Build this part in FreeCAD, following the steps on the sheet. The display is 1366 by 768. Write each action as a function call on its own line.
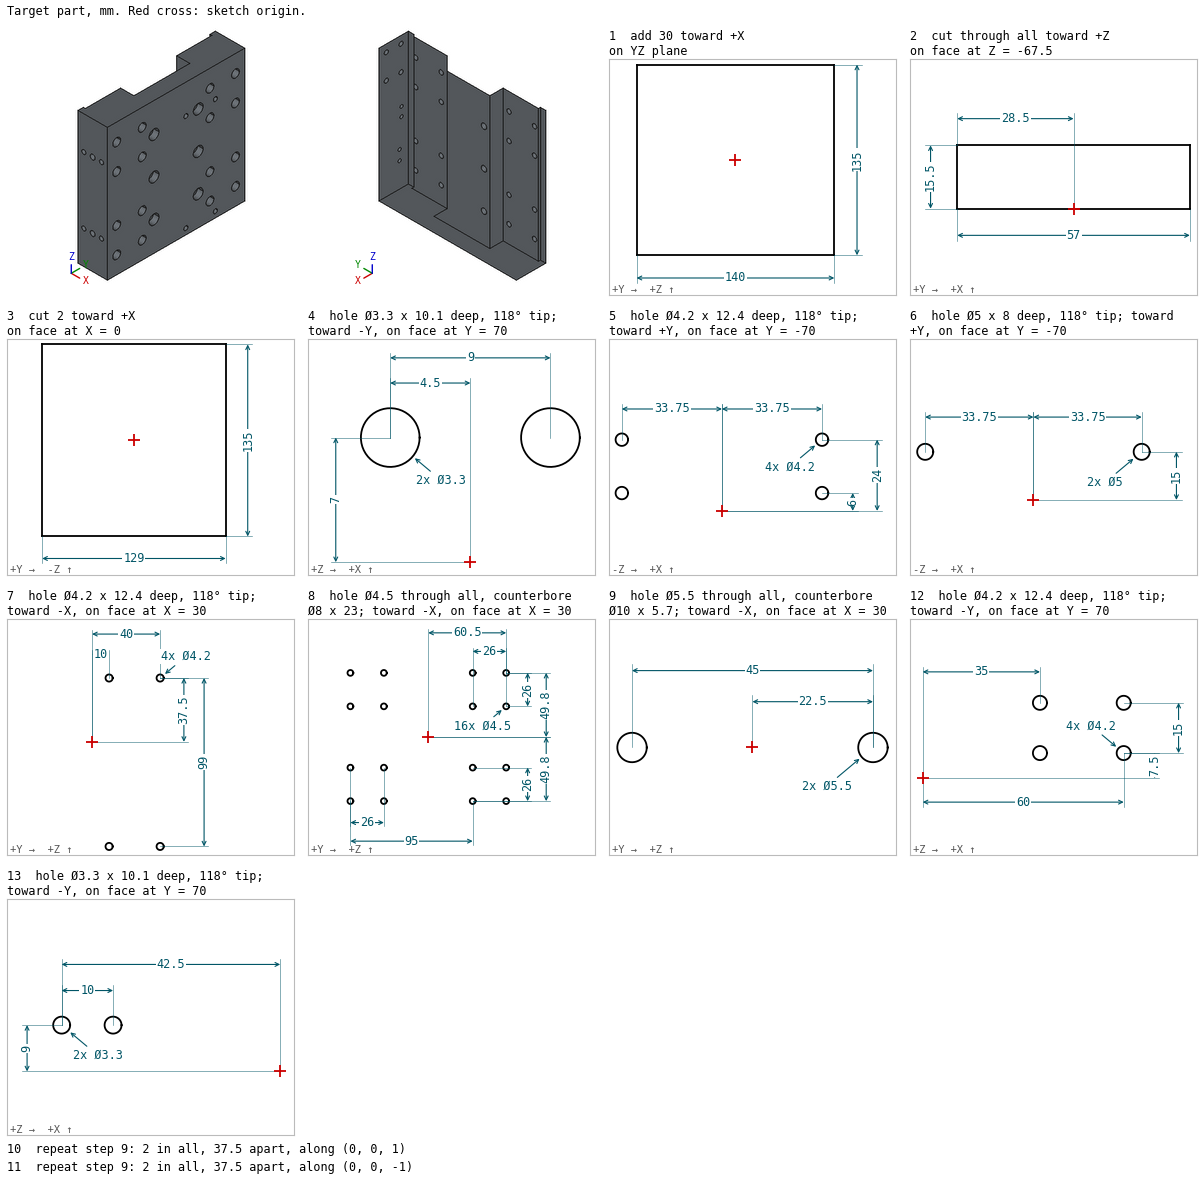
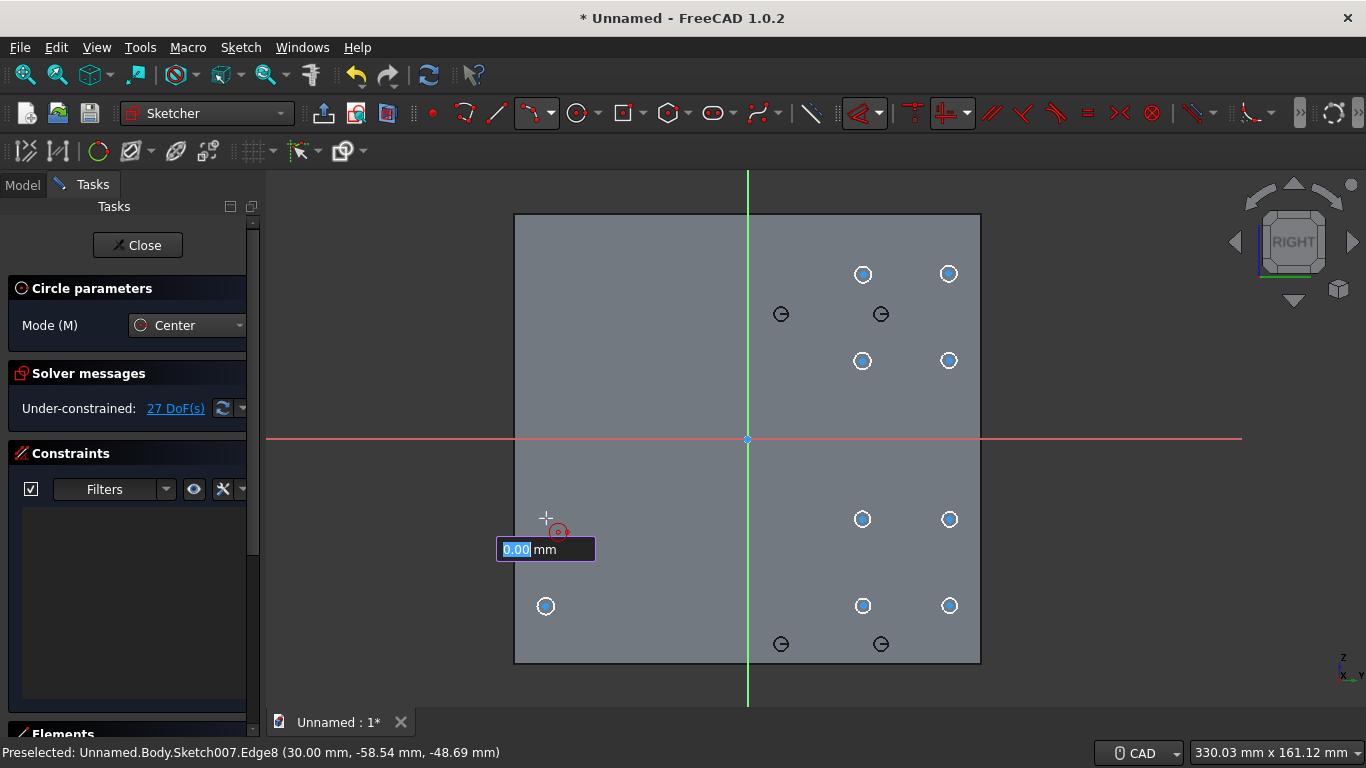
scroll(551, 513, up, 4)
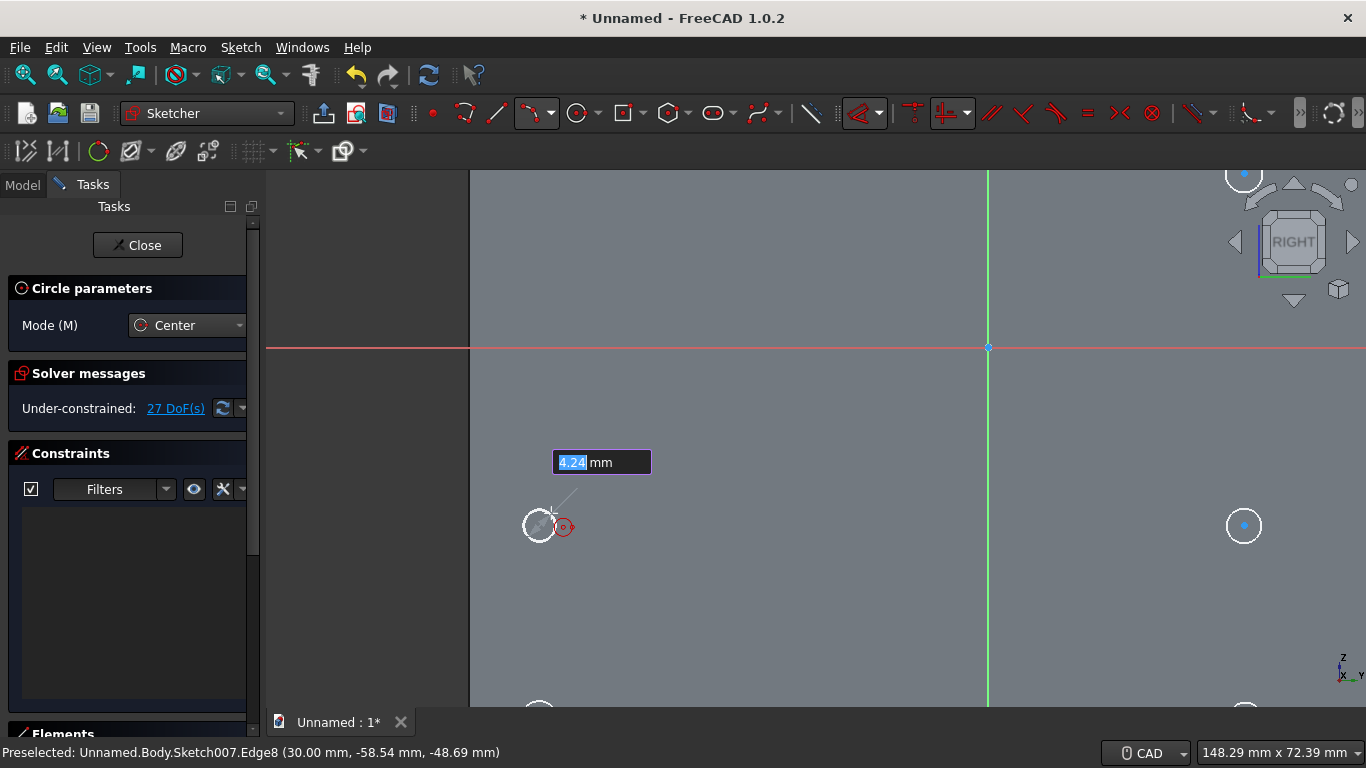
click(551, 512)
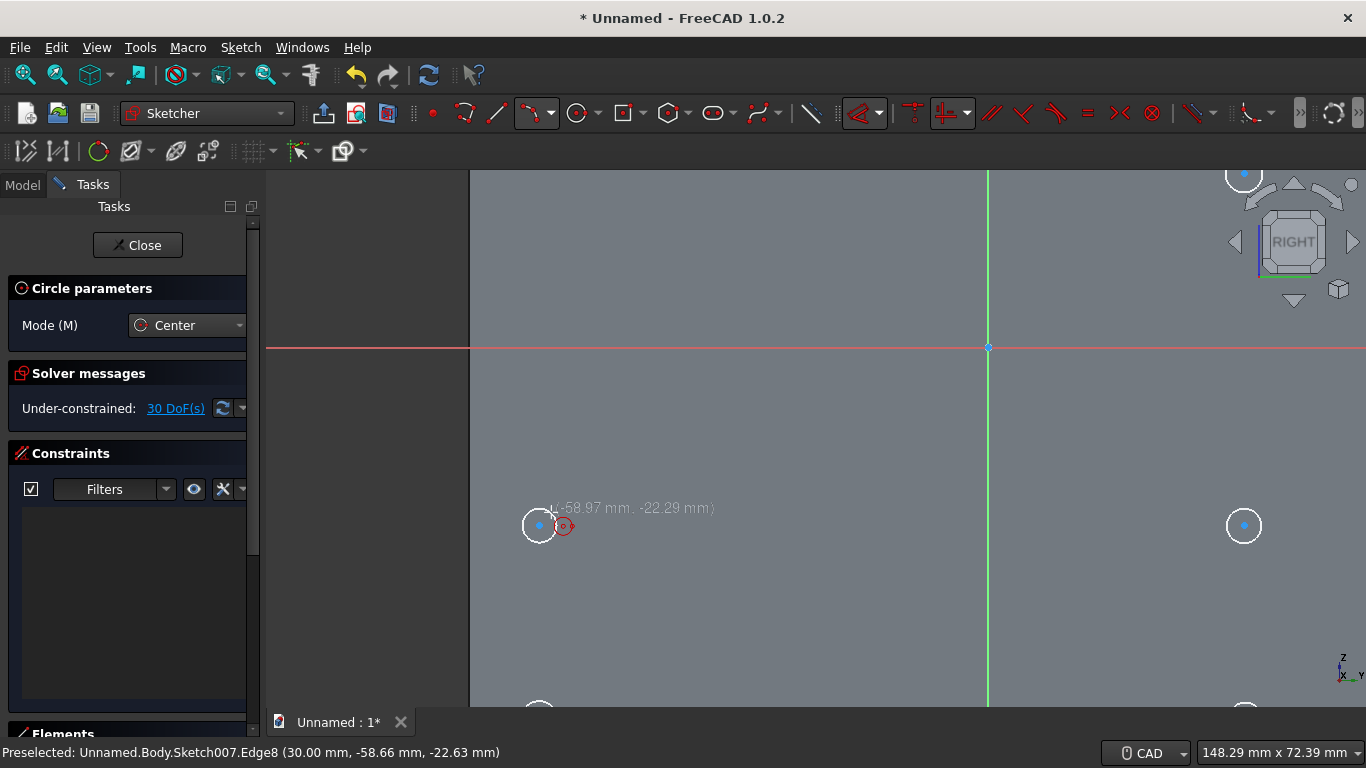
scroll(733, 524, up, 2)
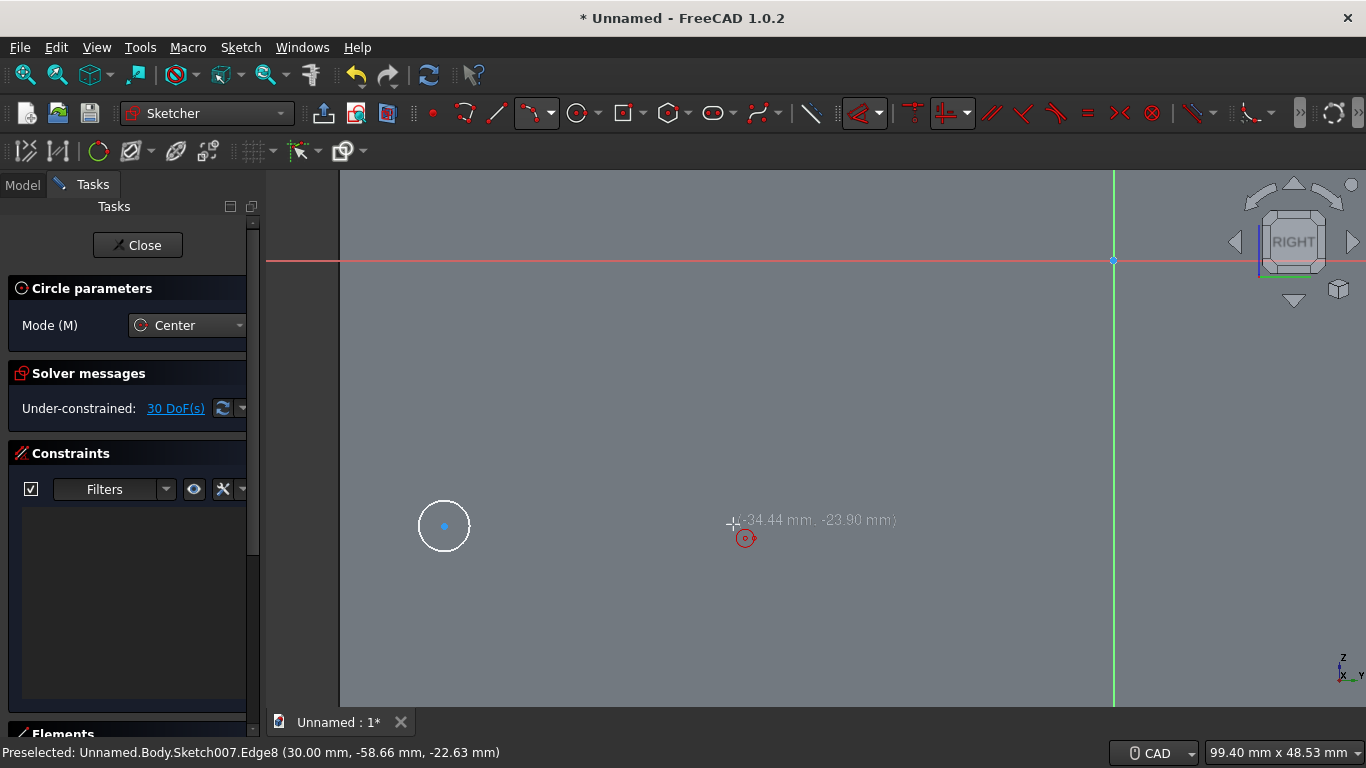
scroll(590, 515, down, 6)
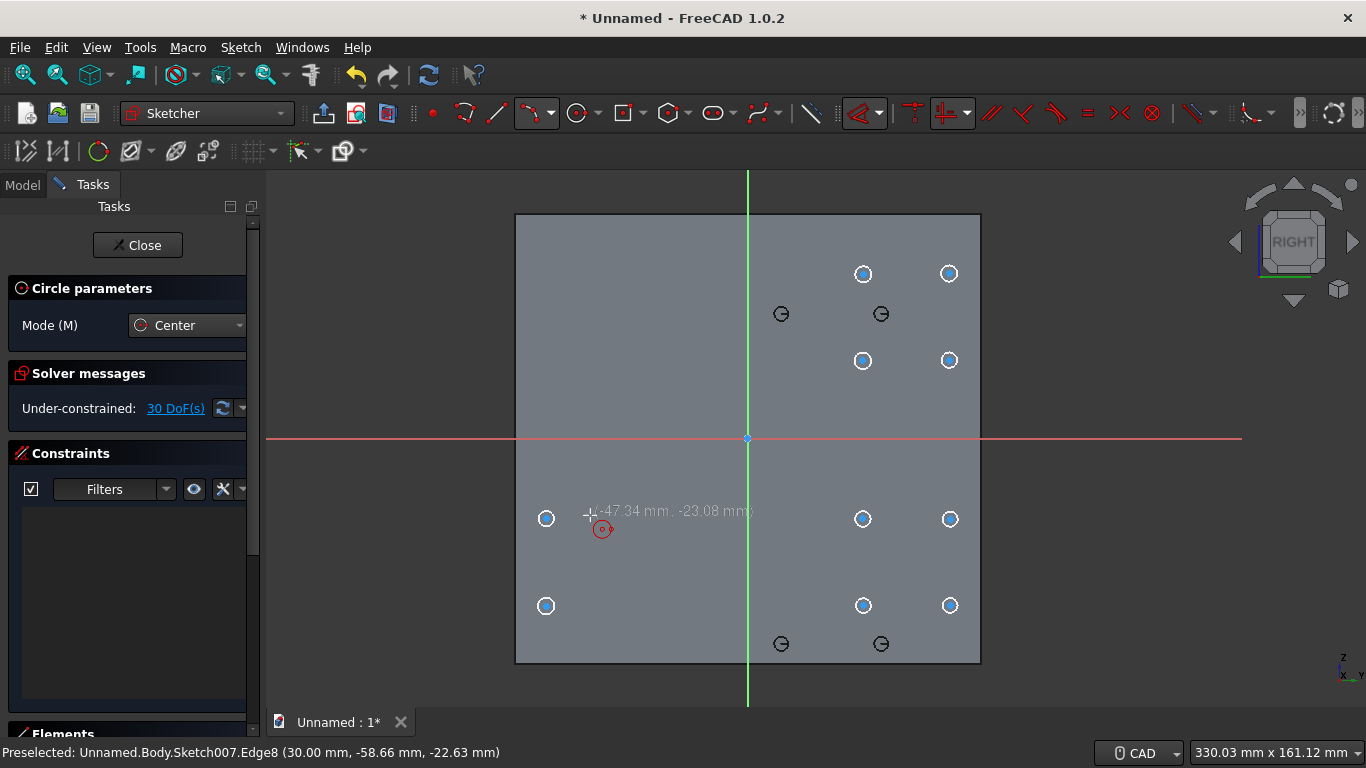
click(633, 518)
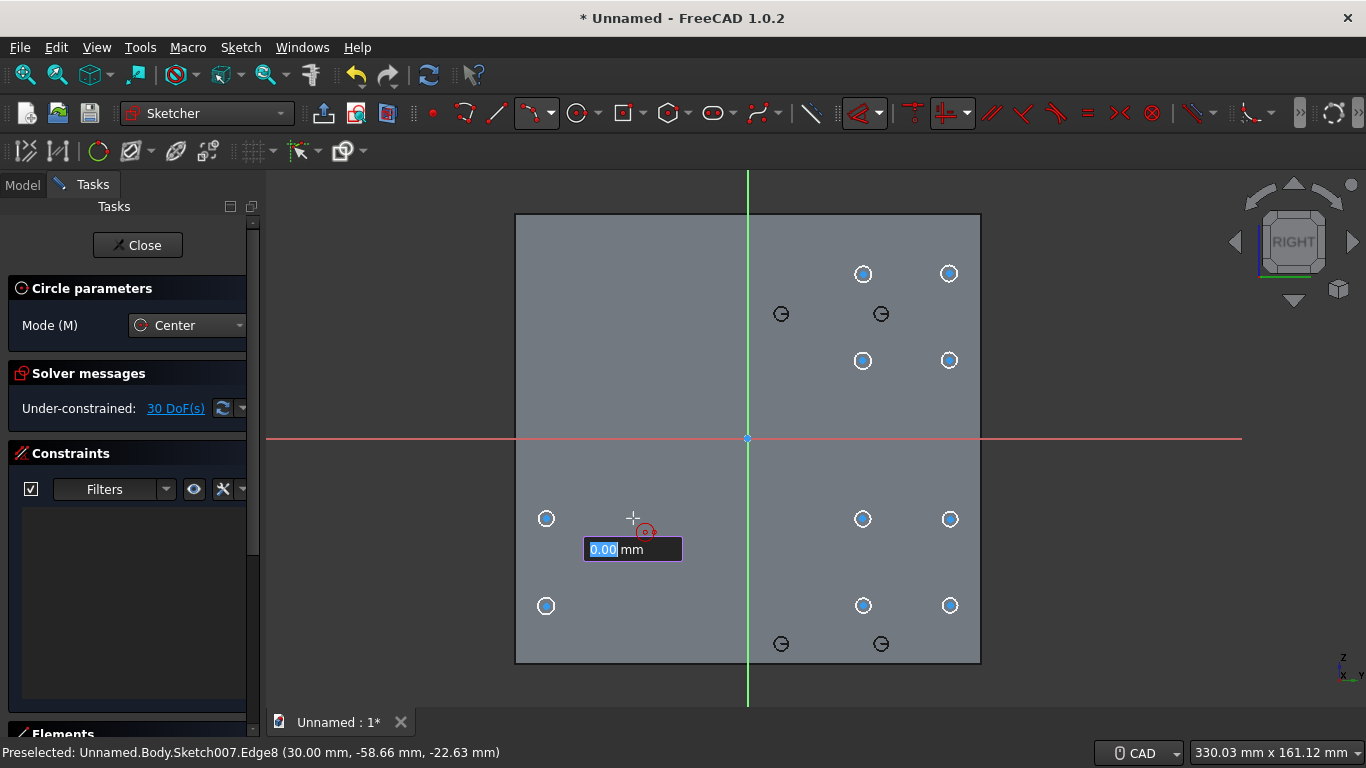
scroll(638, 513, up, 4)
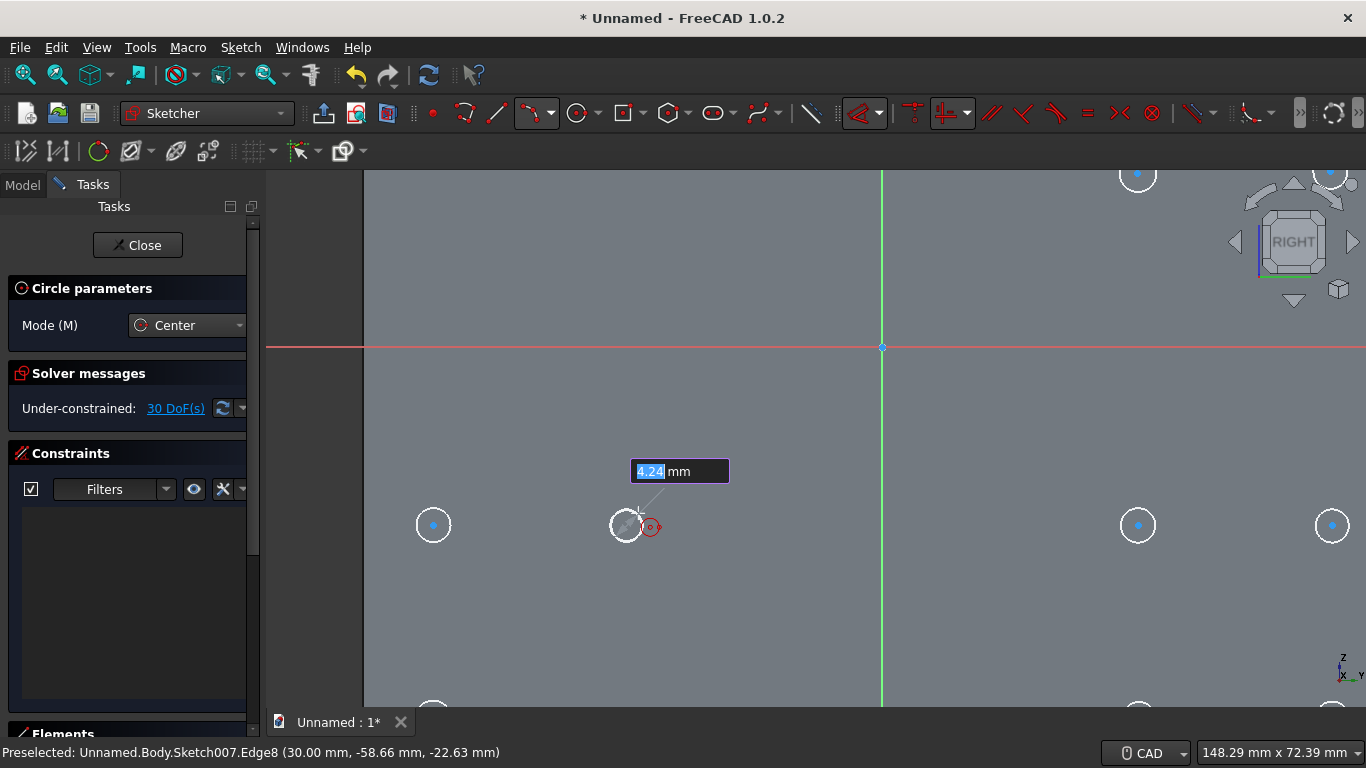
click(638, 512)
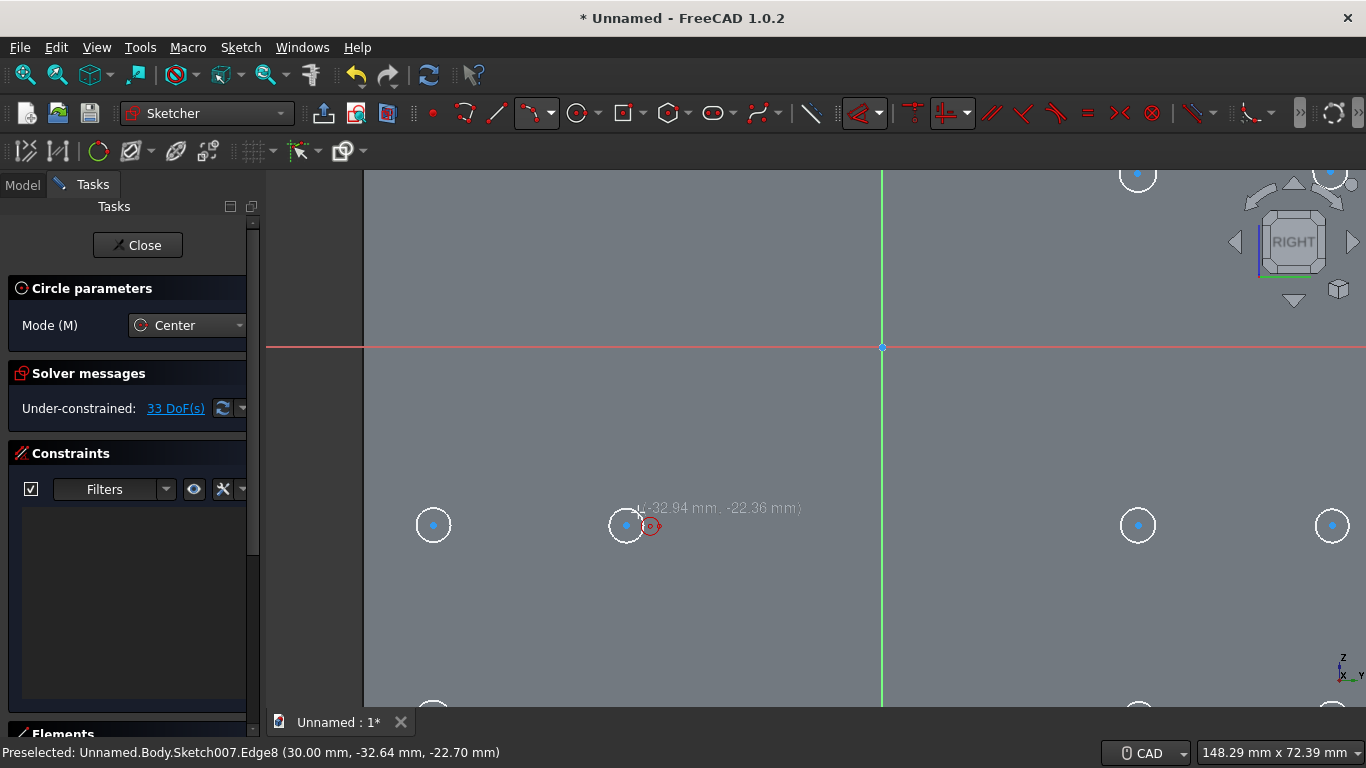
scroll(637, 513, down, 4)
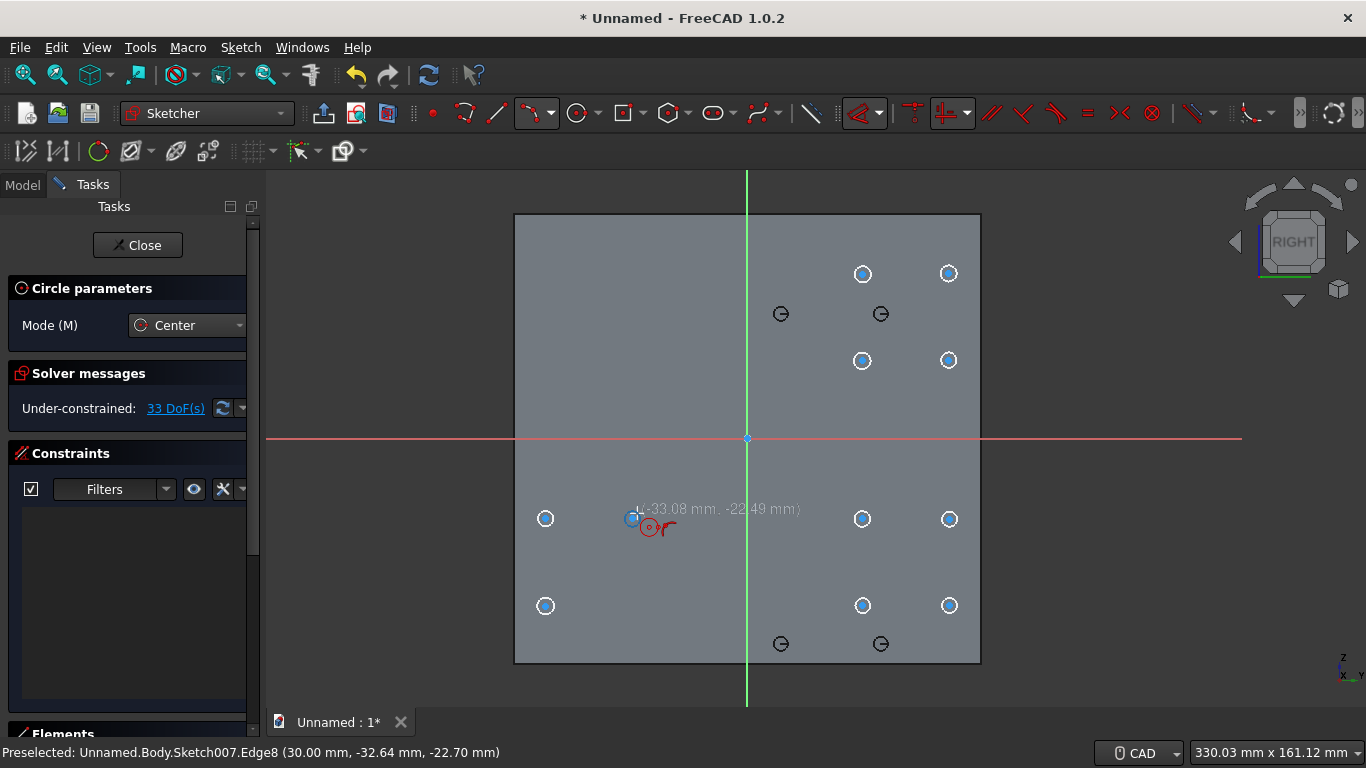
scroll(632, 605, up, 6)